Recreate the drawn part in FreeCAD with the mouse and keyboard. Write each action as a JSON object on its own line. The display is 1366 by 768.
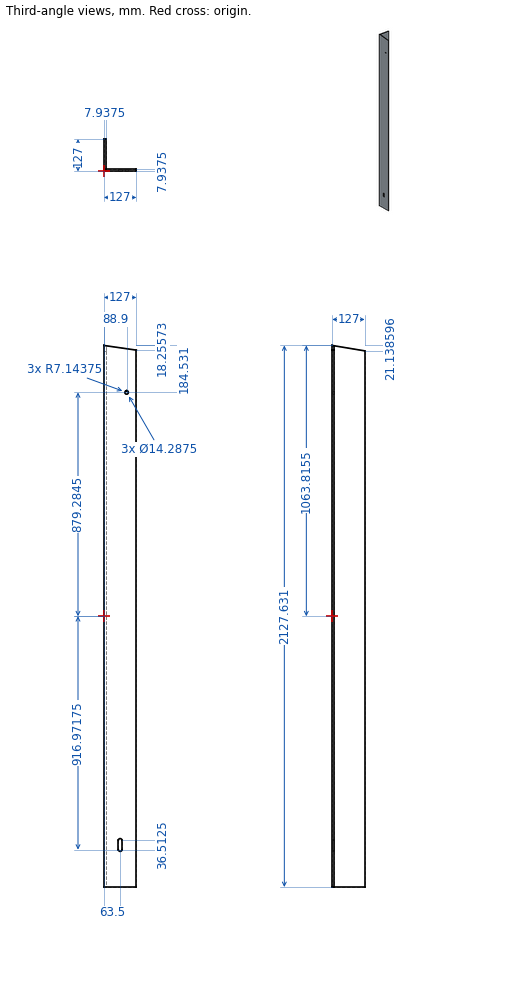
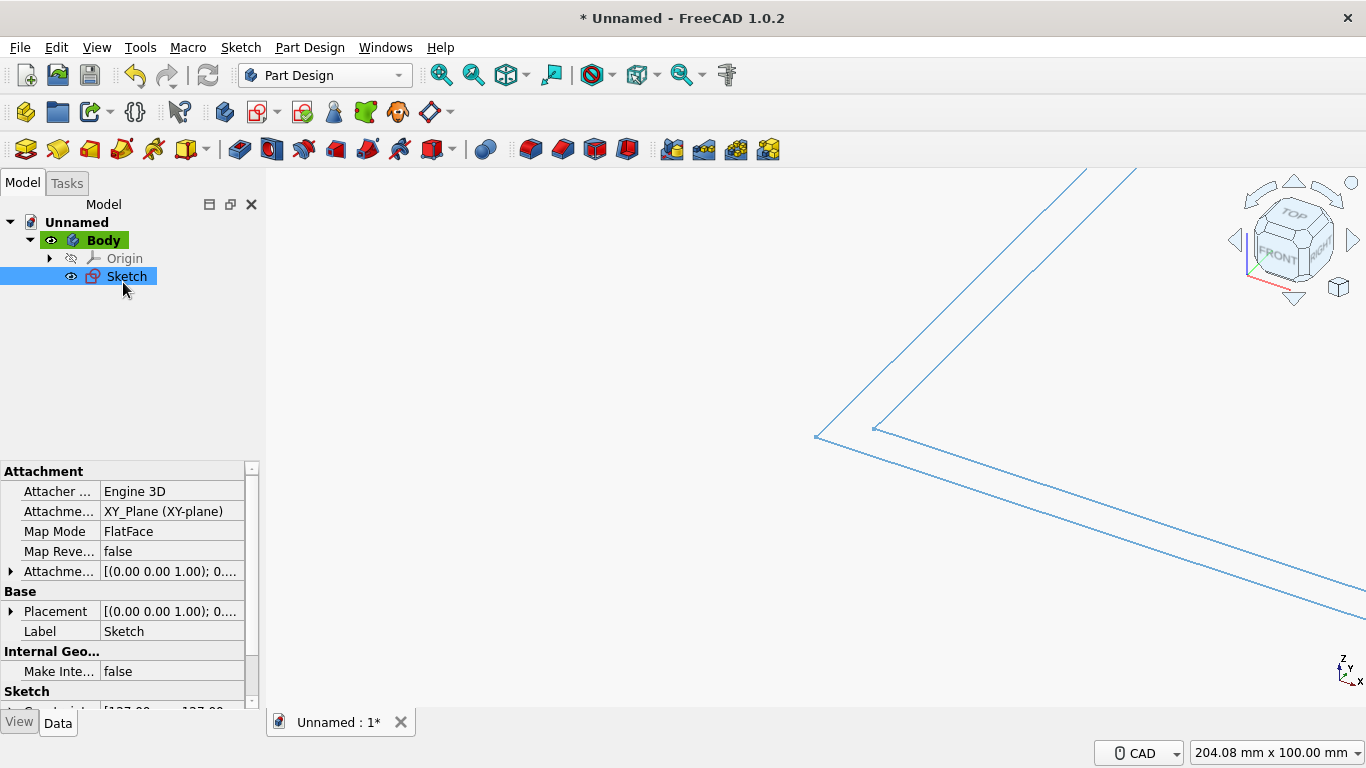
{"action": "left_click", "coordinate": [26, 150]}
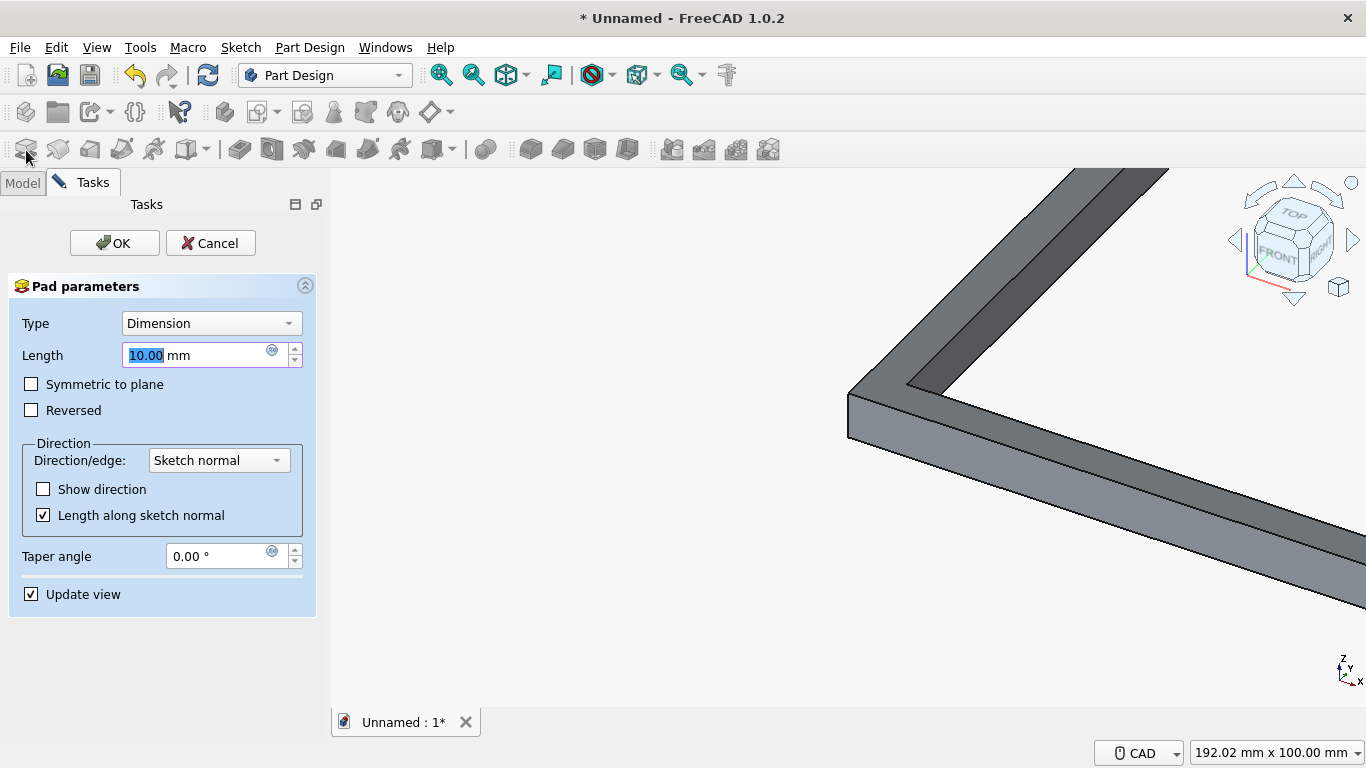
{"action": "type", "text": "2127.631"}
{"action": "key", "text": "Tab"}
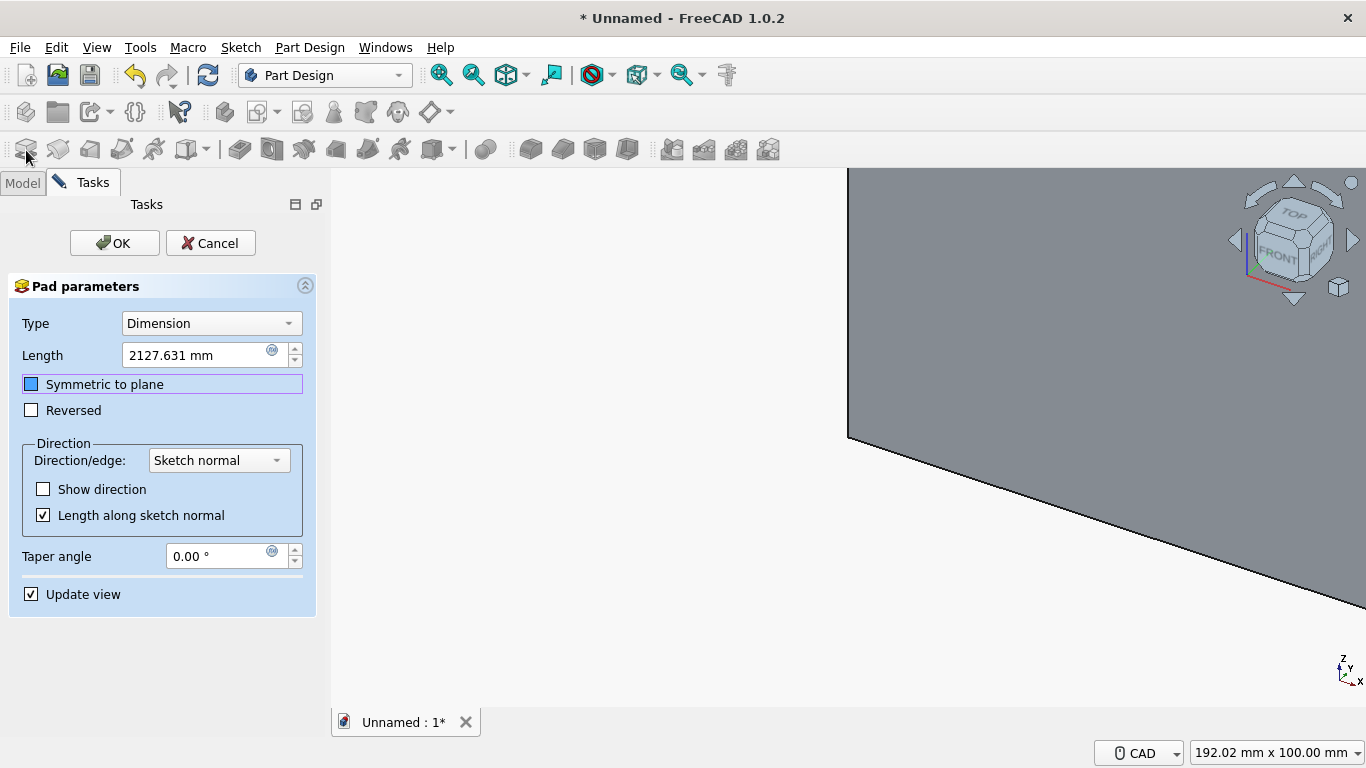
{"action": "left_click", "coordinate": [30, 384]}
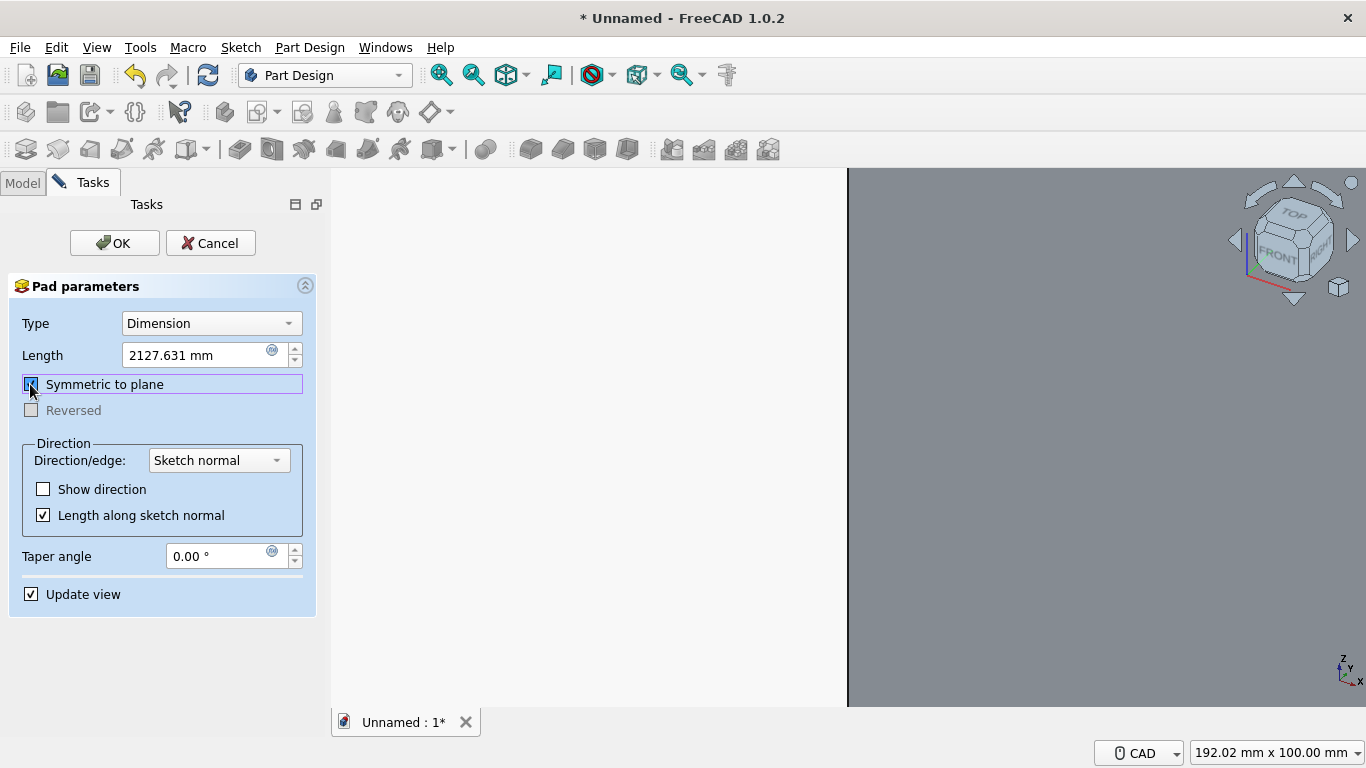
{"action": "left_click", "coordinate": [115, 243]}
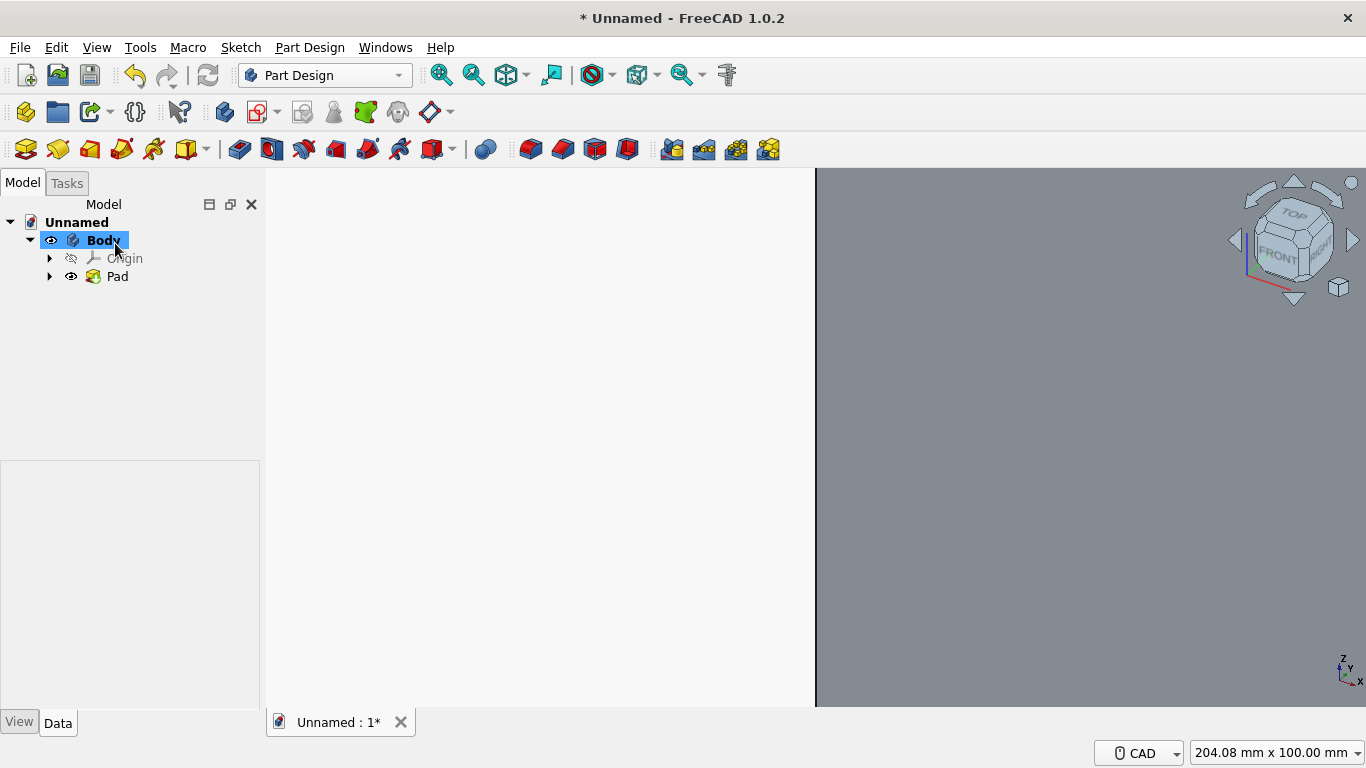
{"action": "key", "text": "v f"}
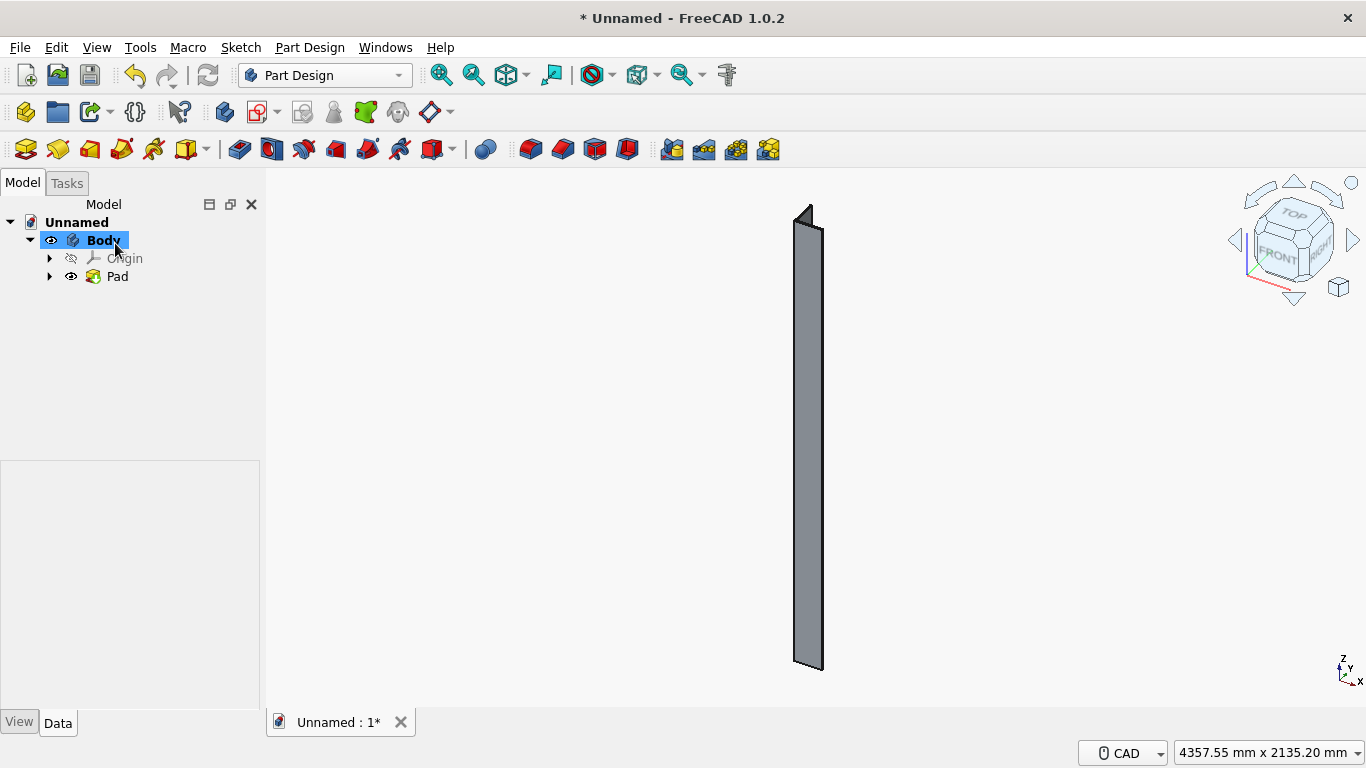
{"action": "left_click", "coordinate": [258, 112]}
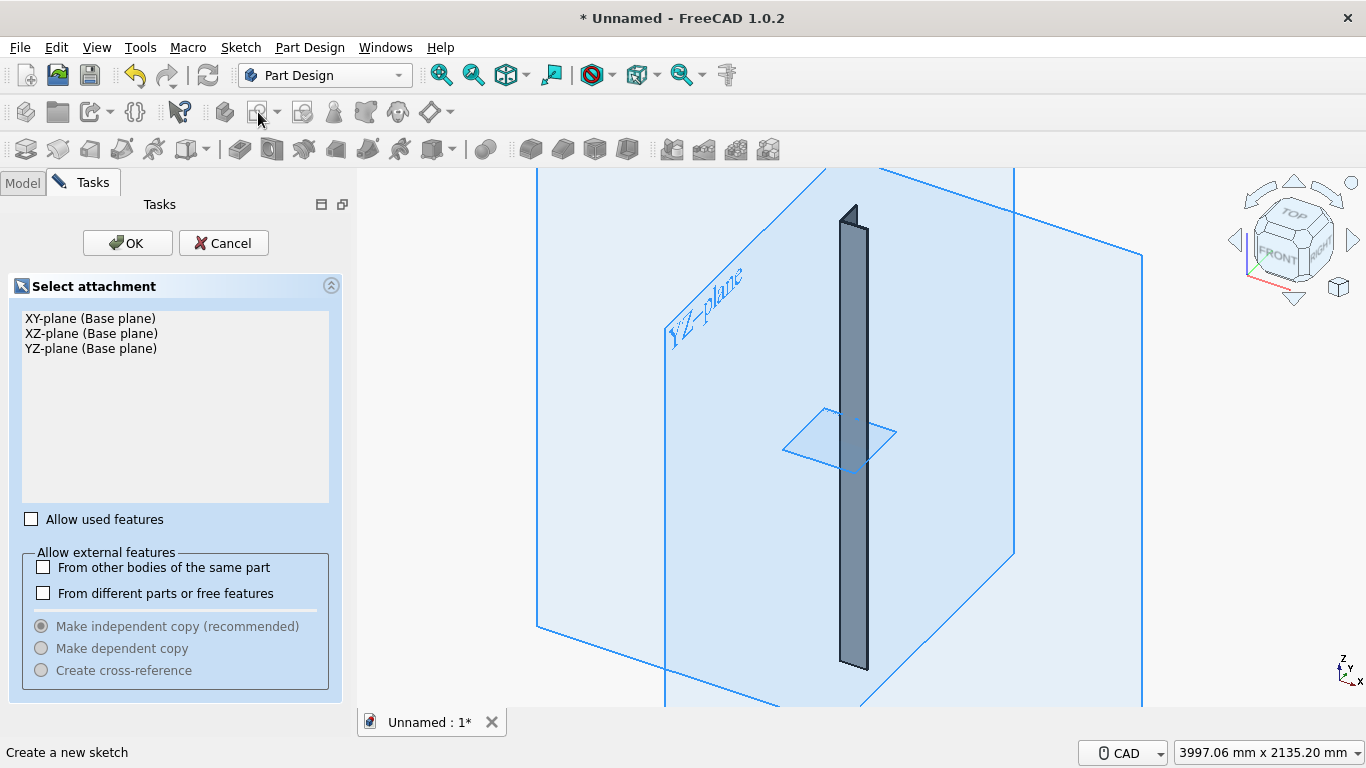
{"action": "left_click", "coordinate": [82, 348]}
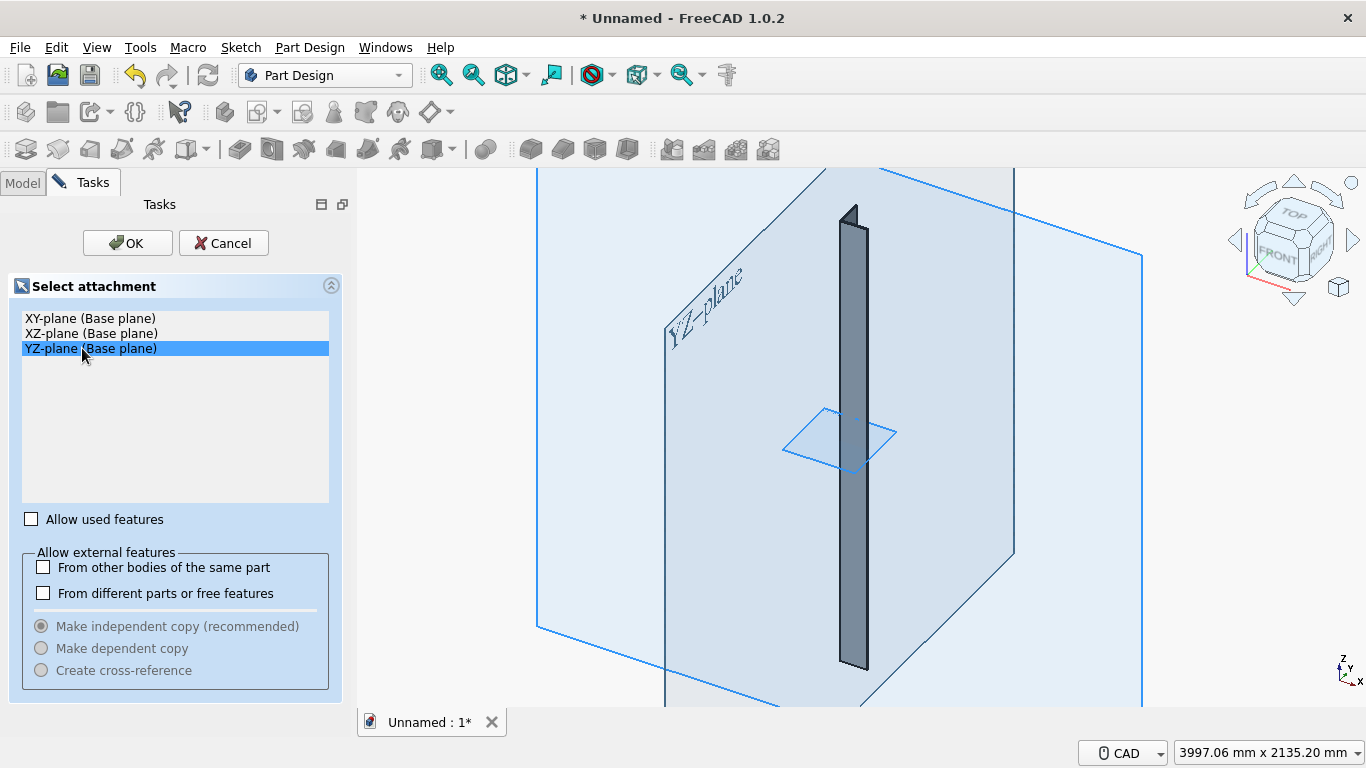
{"action": "left_click", "coordinate": [128, 243]}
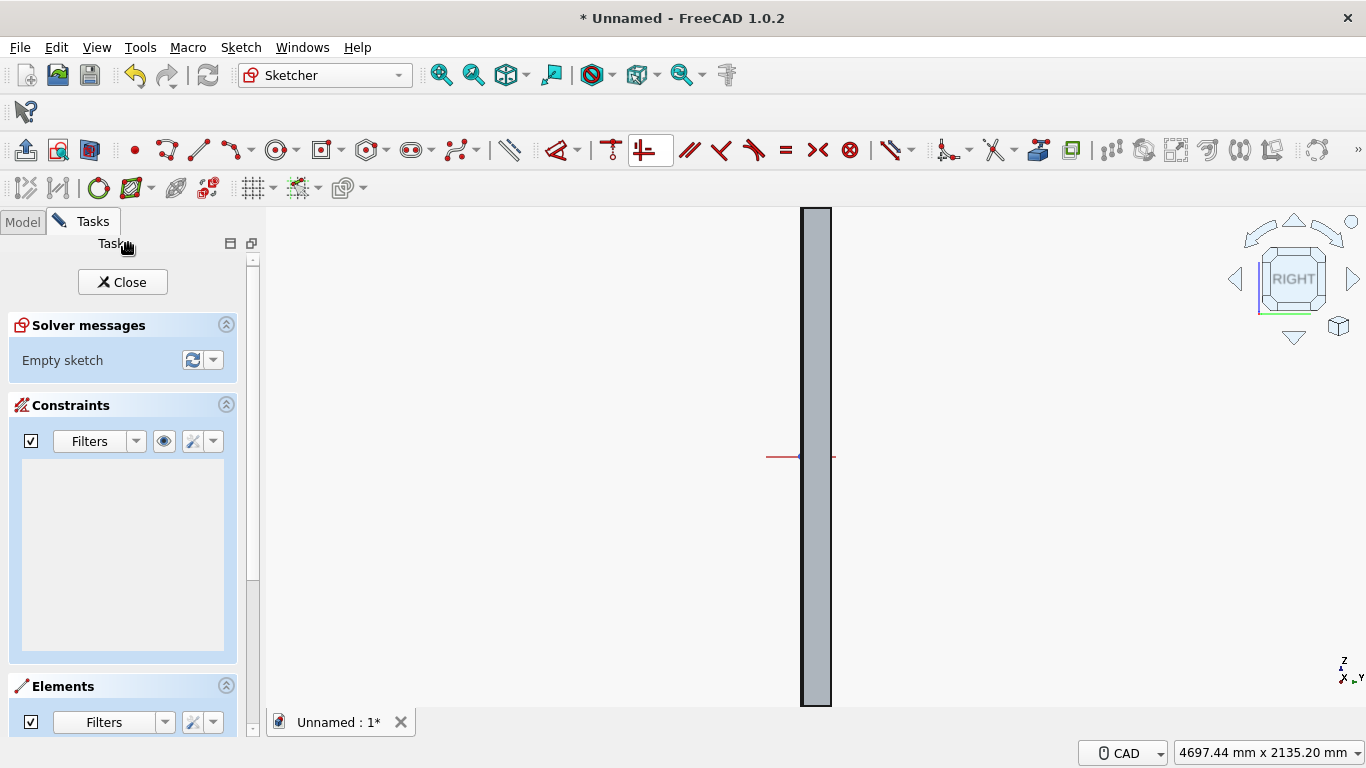
{"action": "key", "text": "q s"}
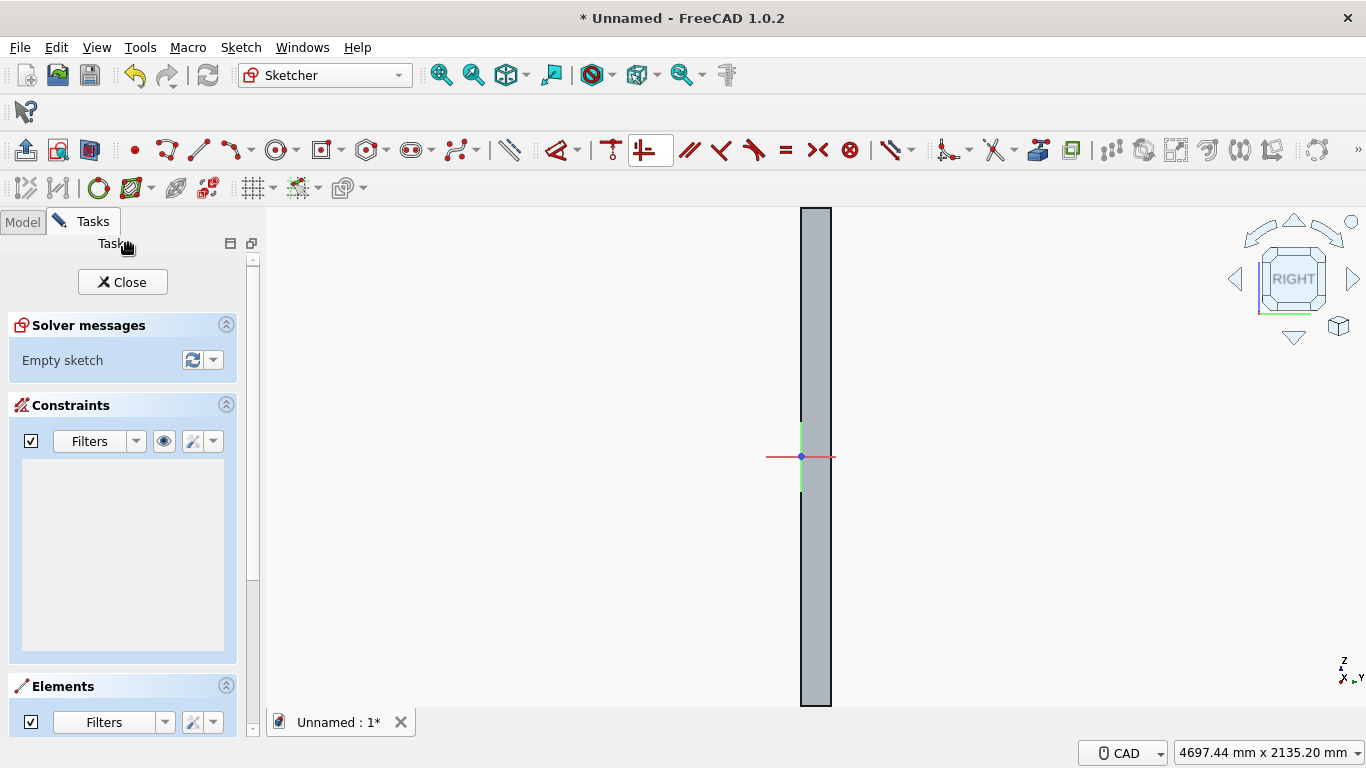
{"action": "scroll", "coordinate": [748, 457], "scroll_direction": "down", "scroll_amount": 5}